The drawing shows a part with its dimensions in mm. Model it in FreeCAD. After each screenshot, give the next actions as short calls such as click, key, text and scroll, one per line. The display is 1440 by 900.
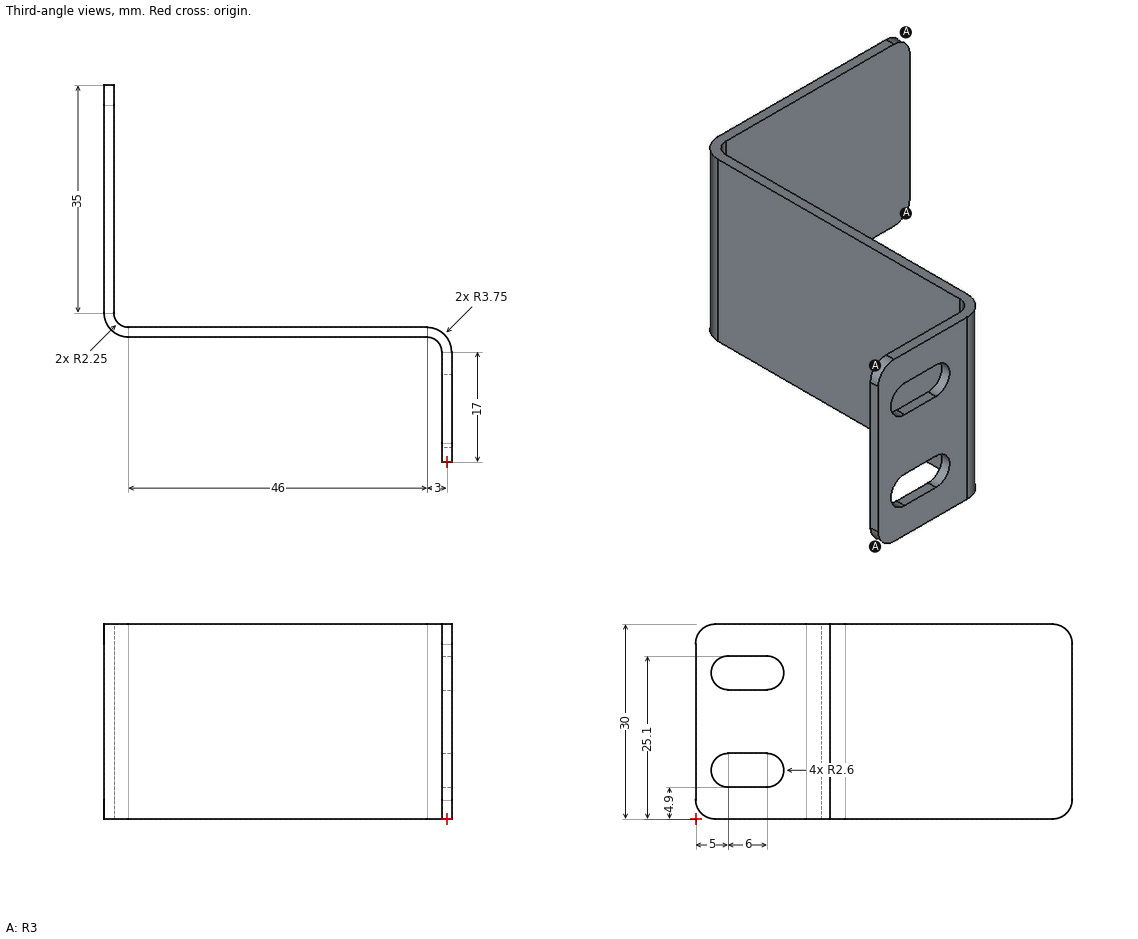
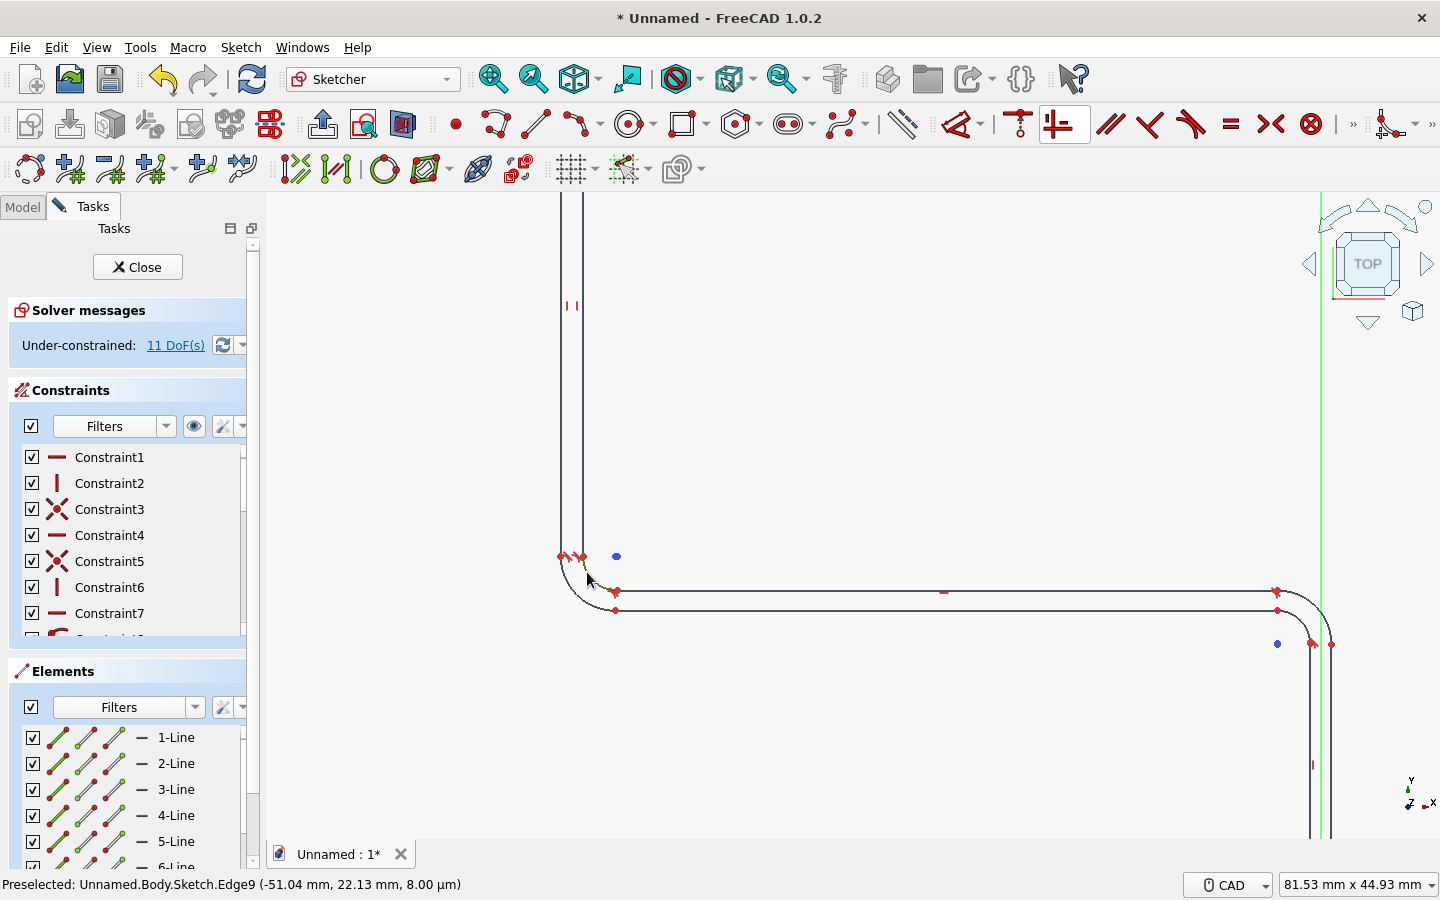
click(567, 581)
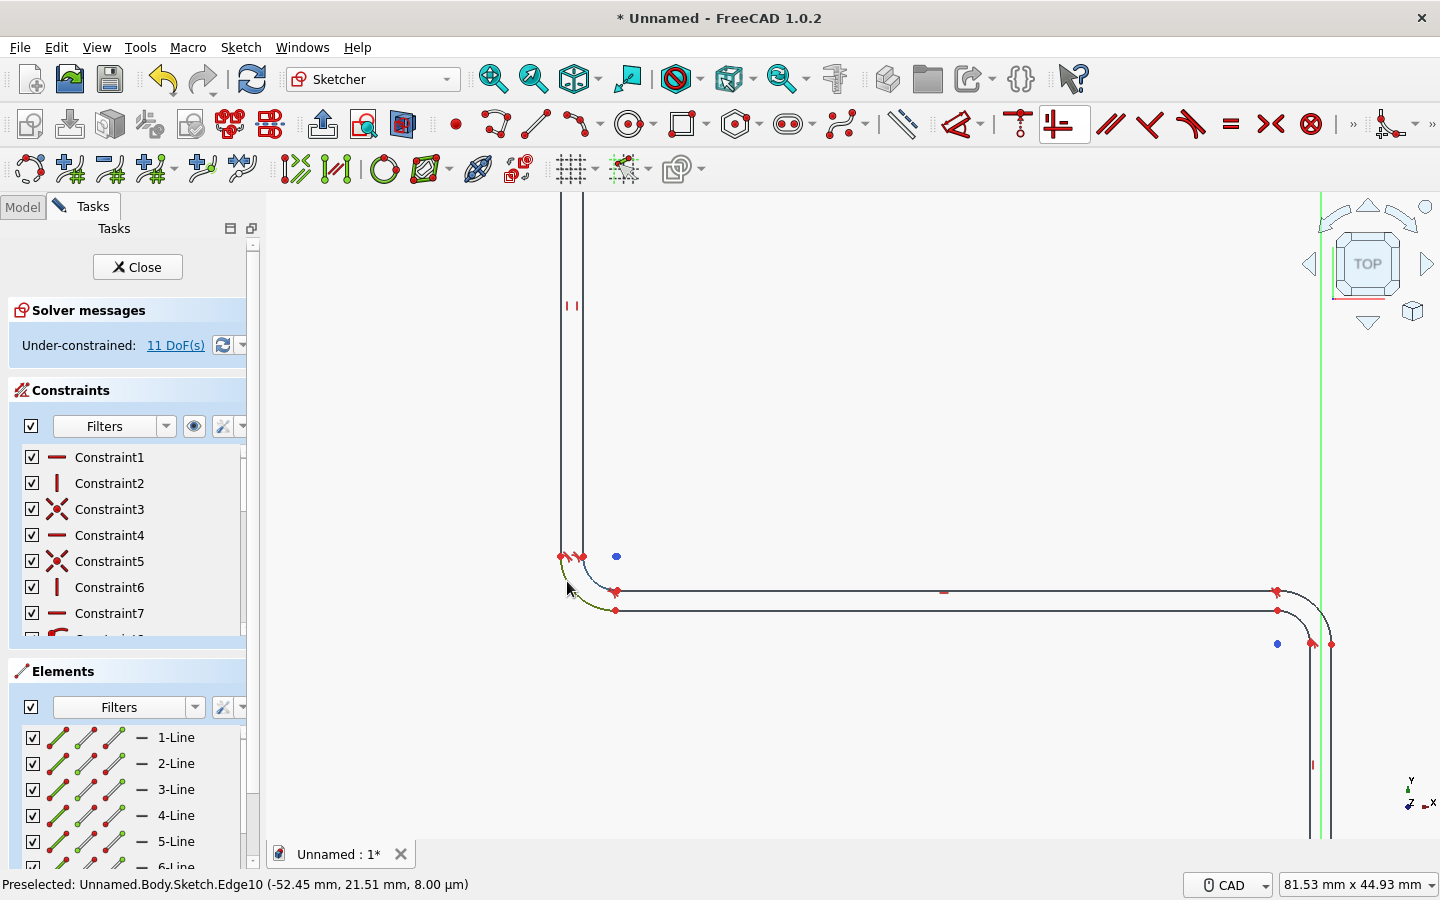
key(c)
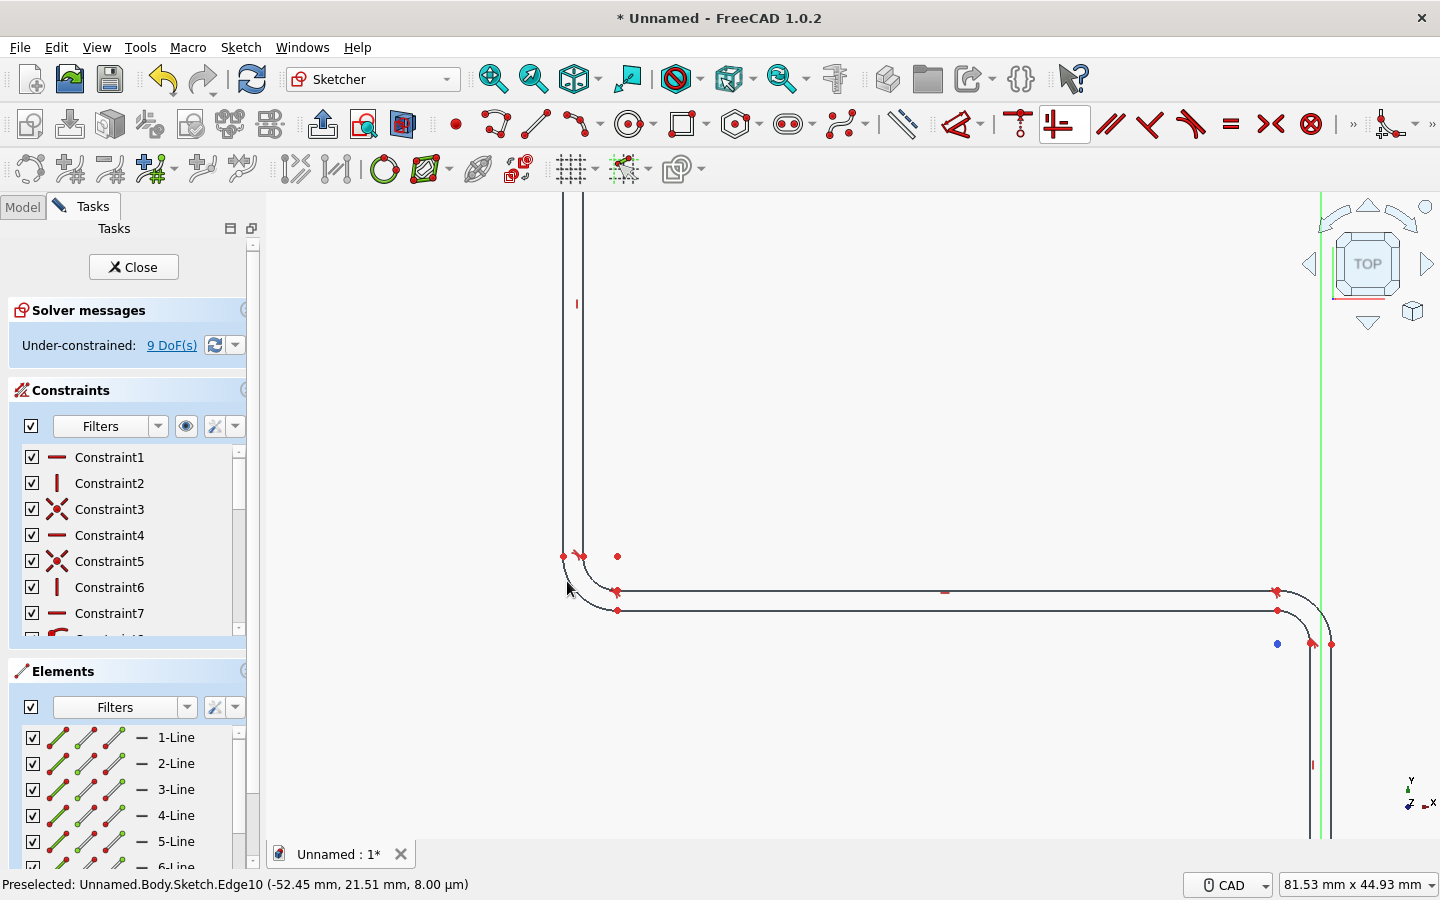
scroll(588, 571, down, 3)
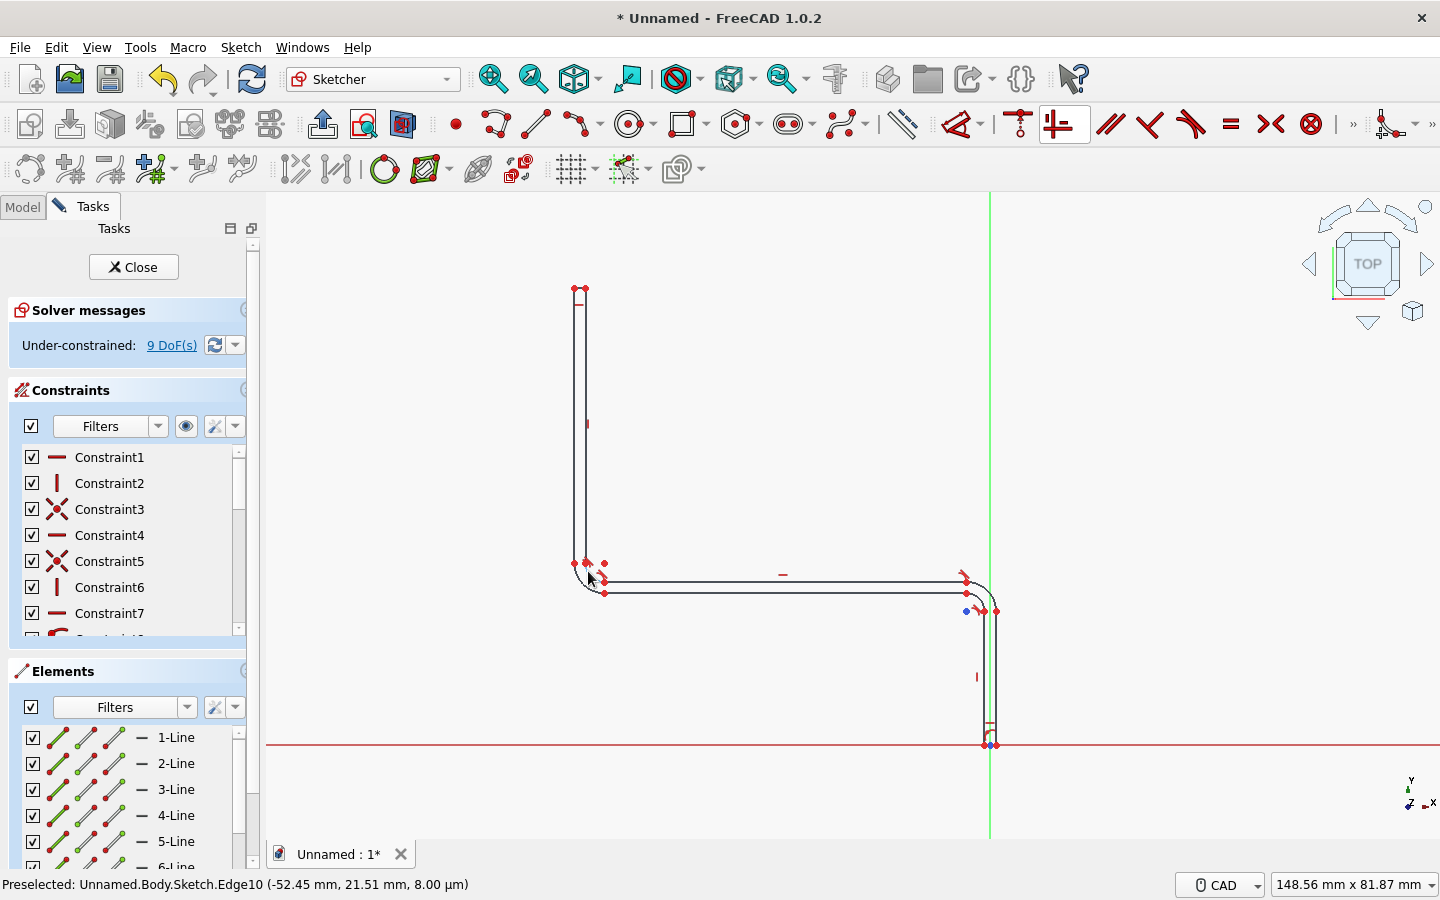
scroll(982, 603, up, 3)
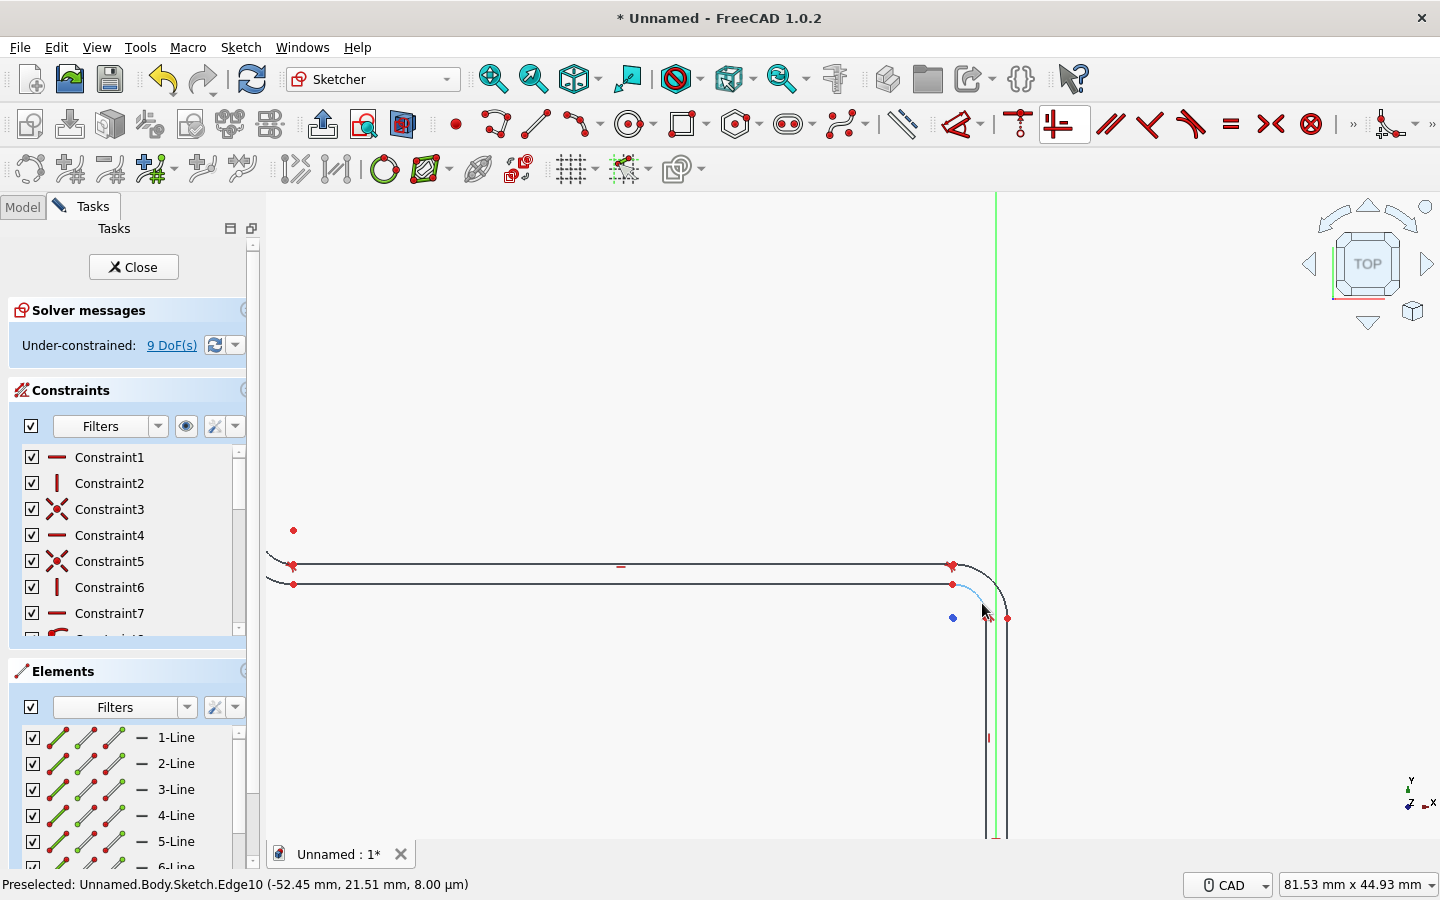
click(982, 602)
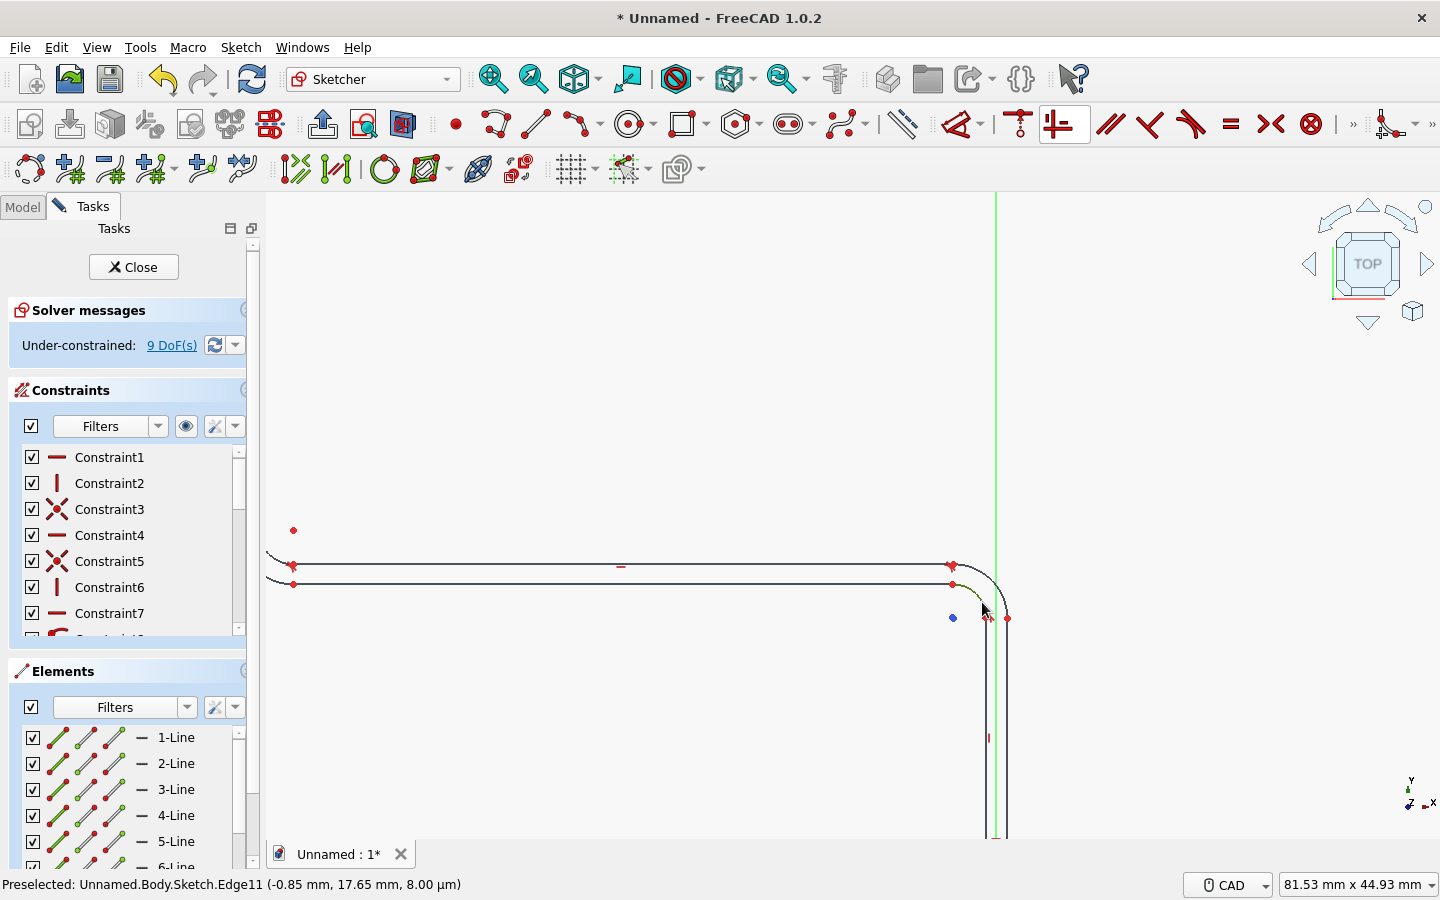
click(978, 570)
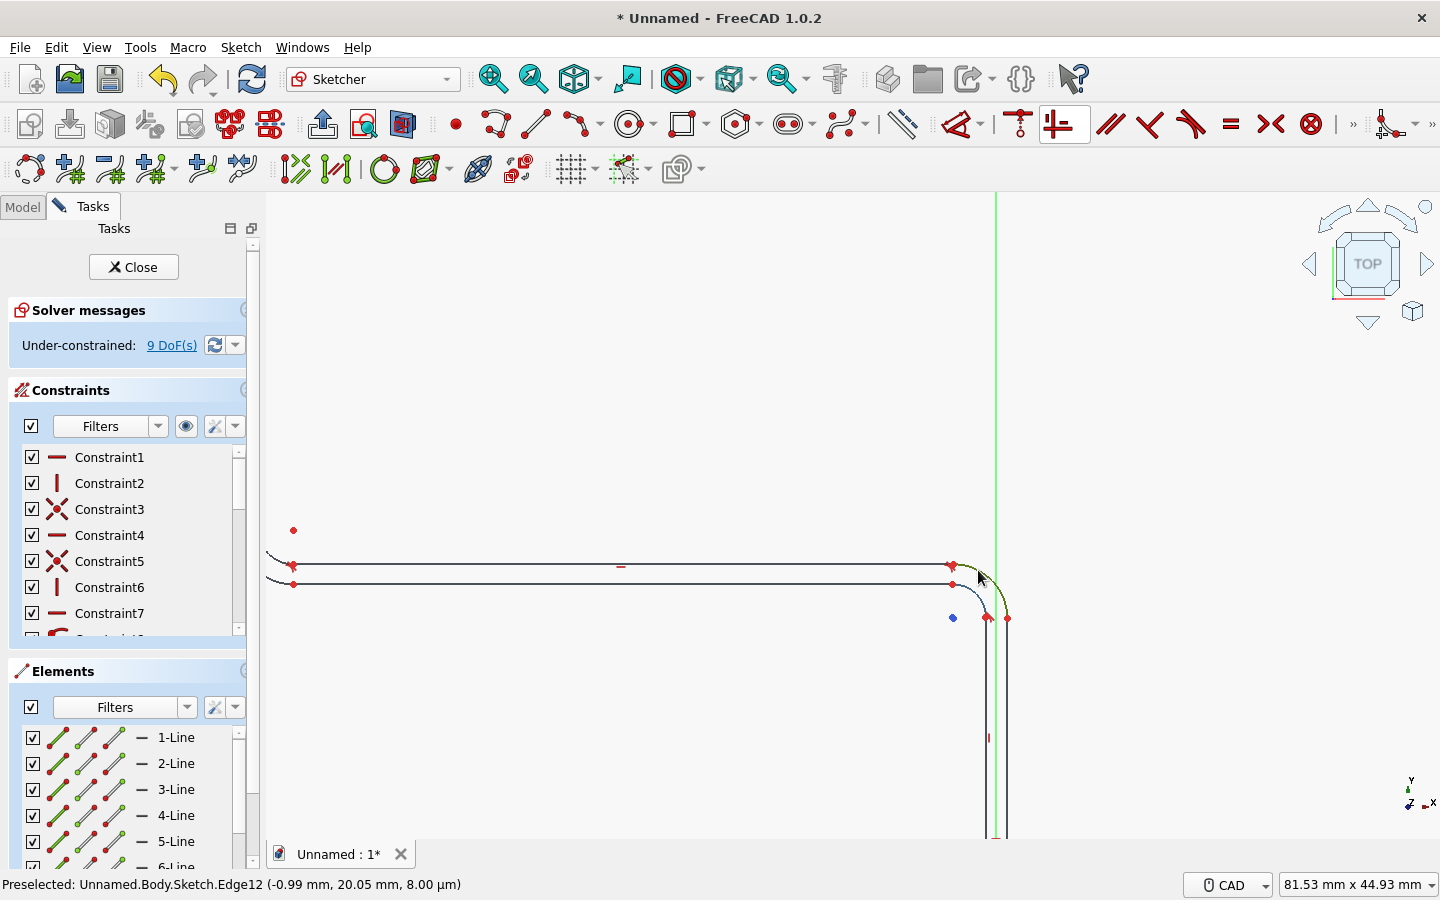
click(1018, 124)